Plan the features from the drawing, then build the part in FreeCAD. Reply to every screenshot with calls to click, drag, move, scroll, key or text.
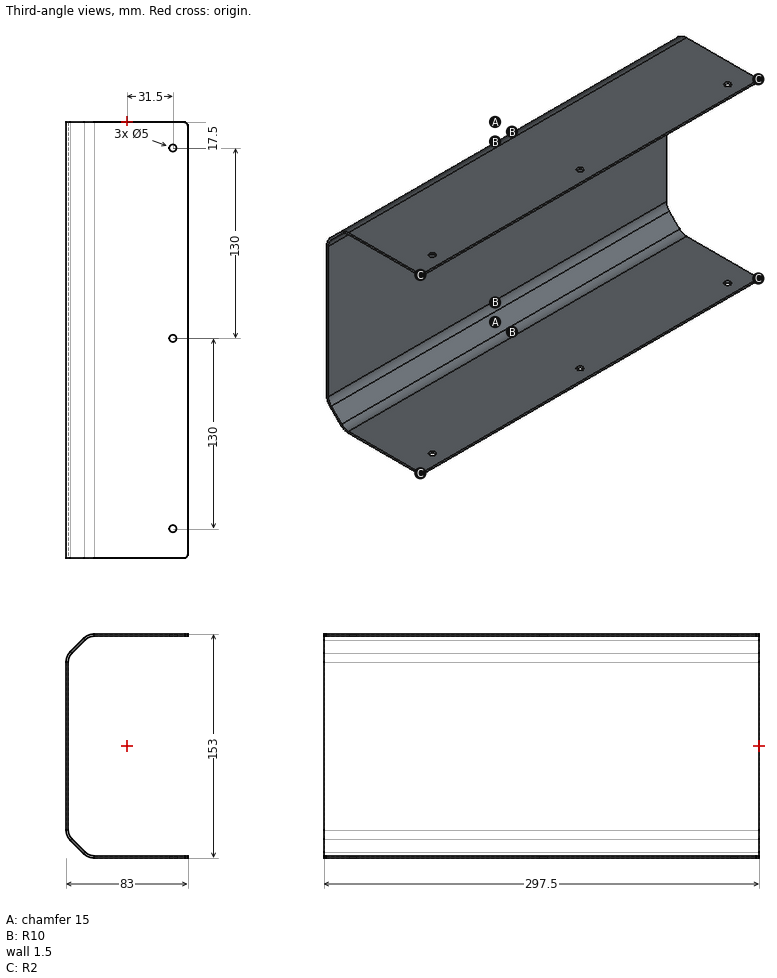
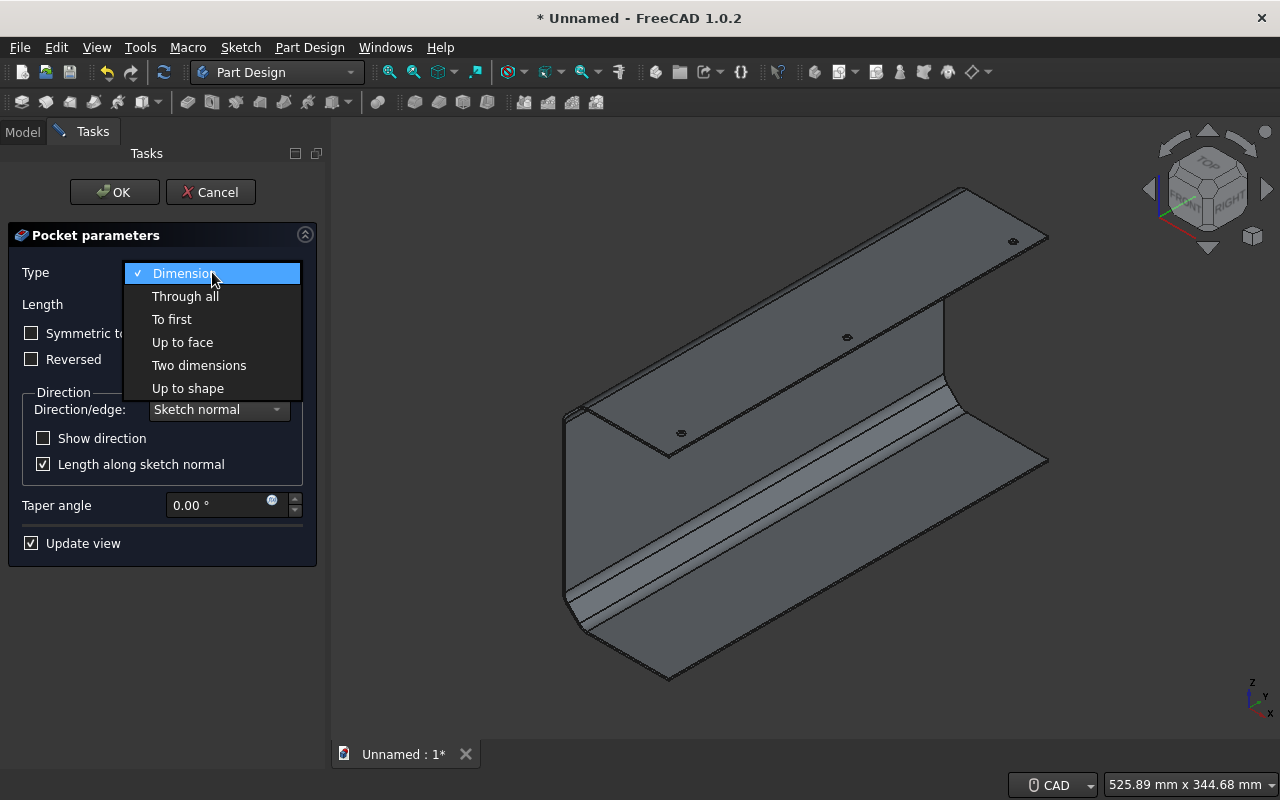
click(212, 296)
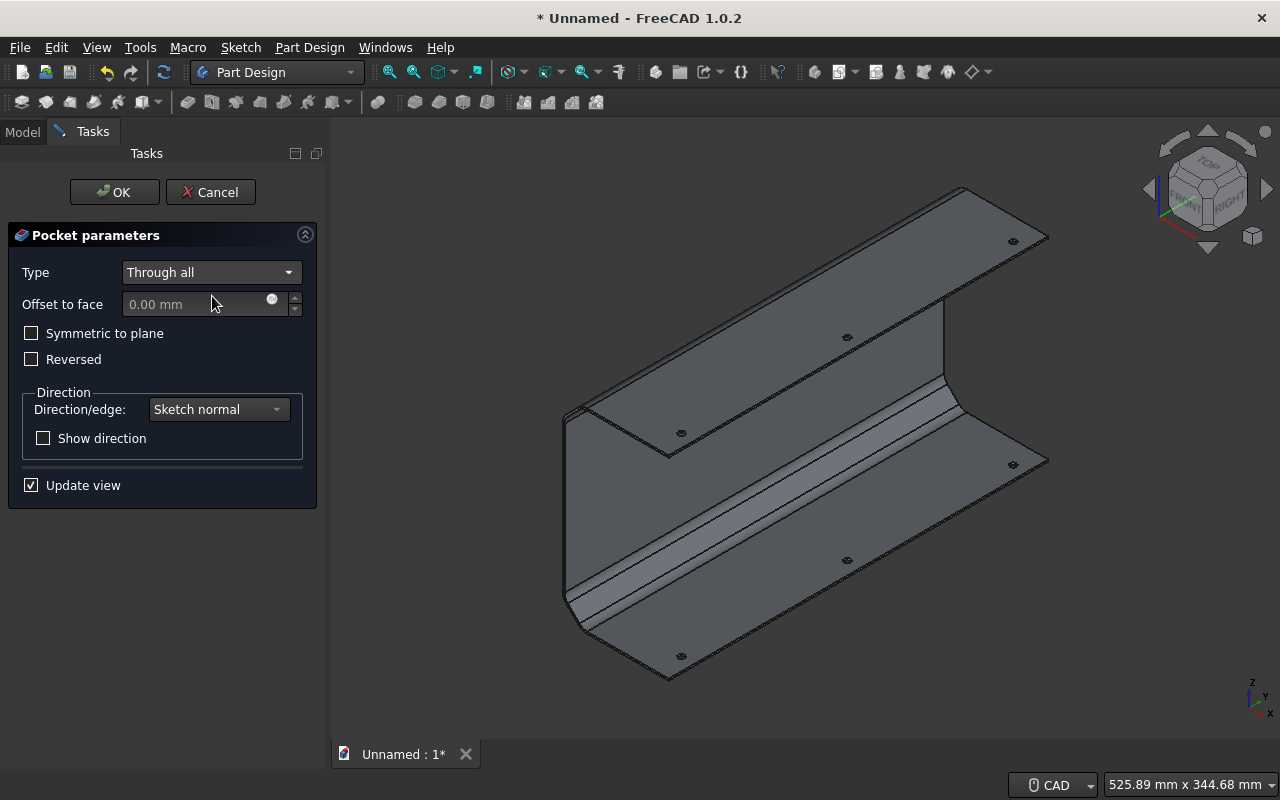
click(115, 192)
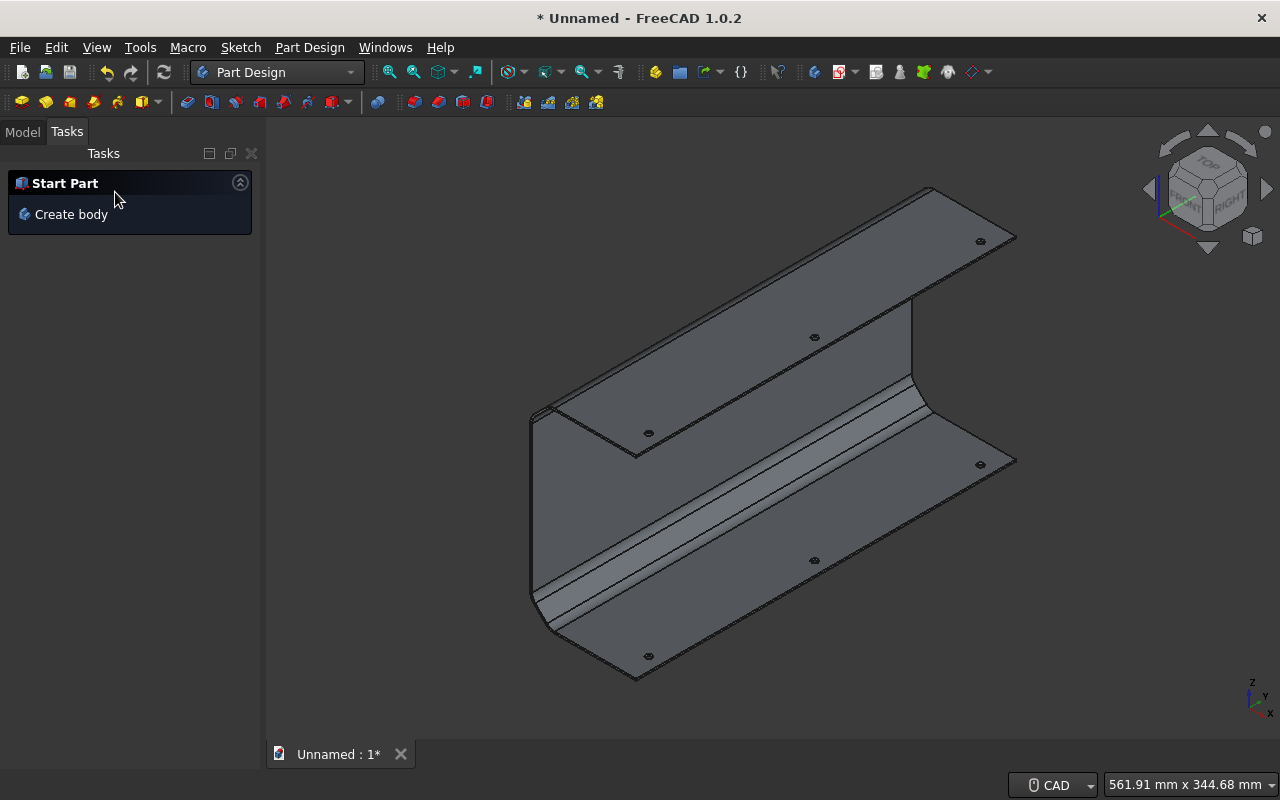
scroll(636, 456, up, 14)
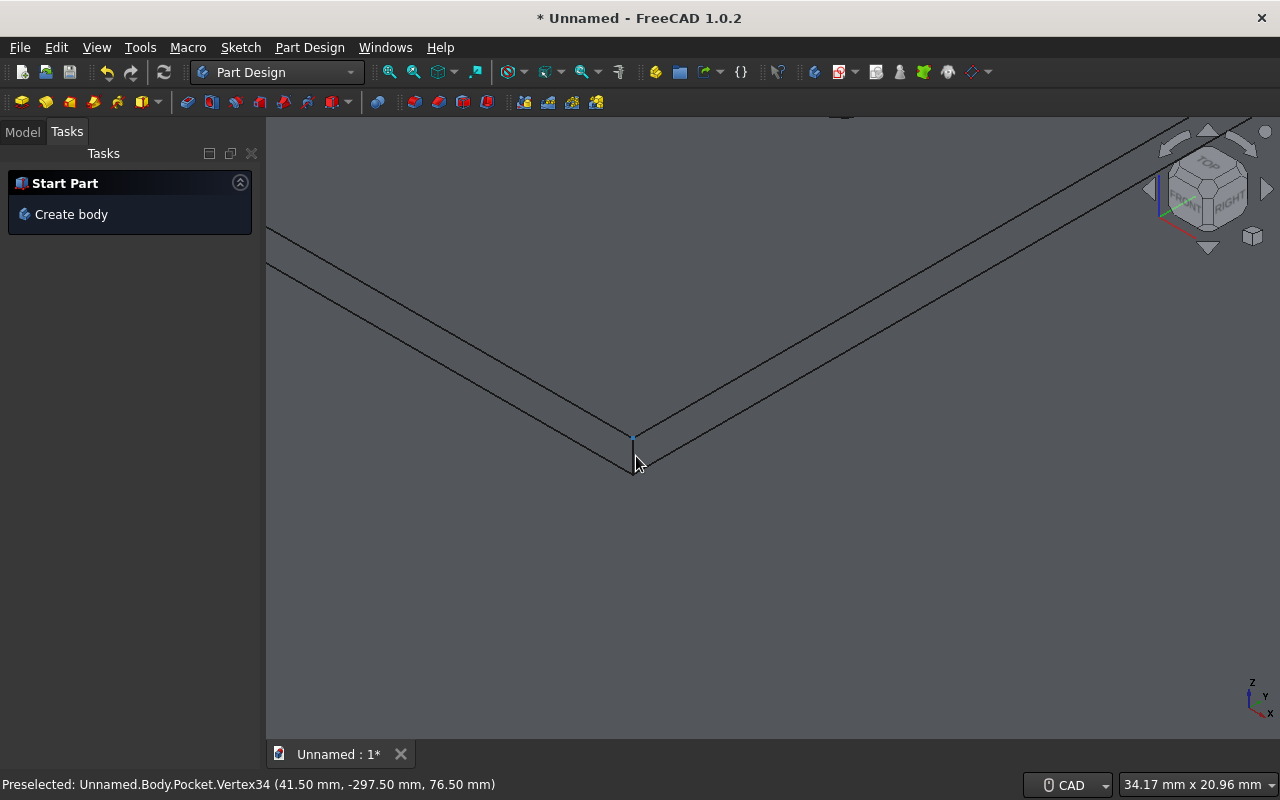
click(633, 456)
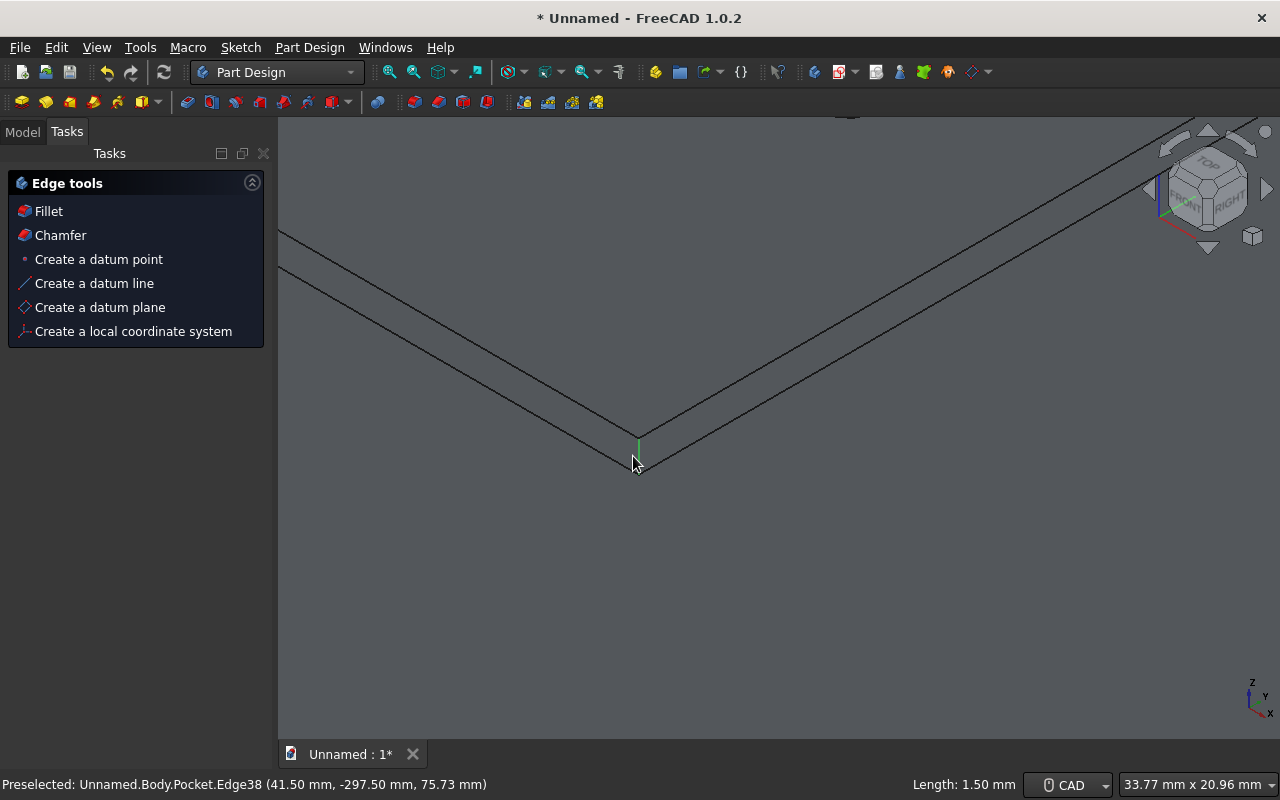
key(v)
key(f)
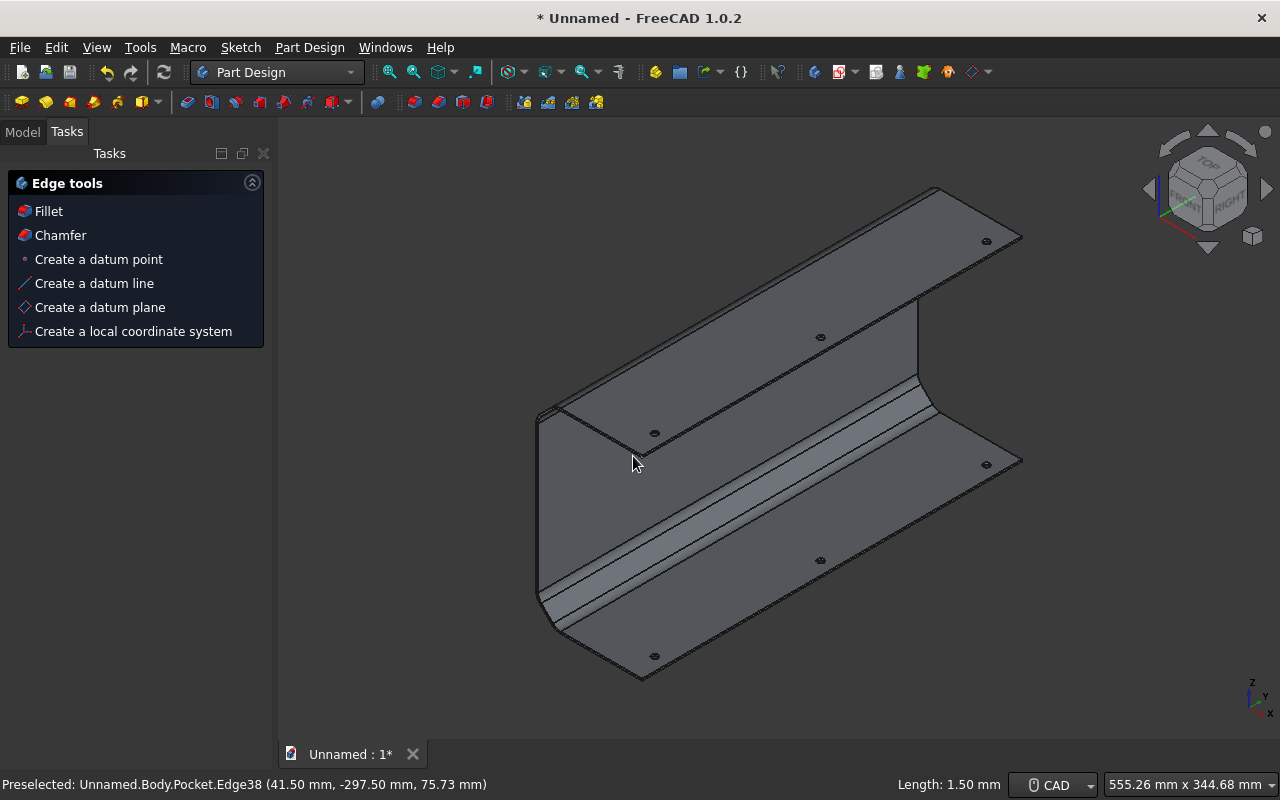
key(2)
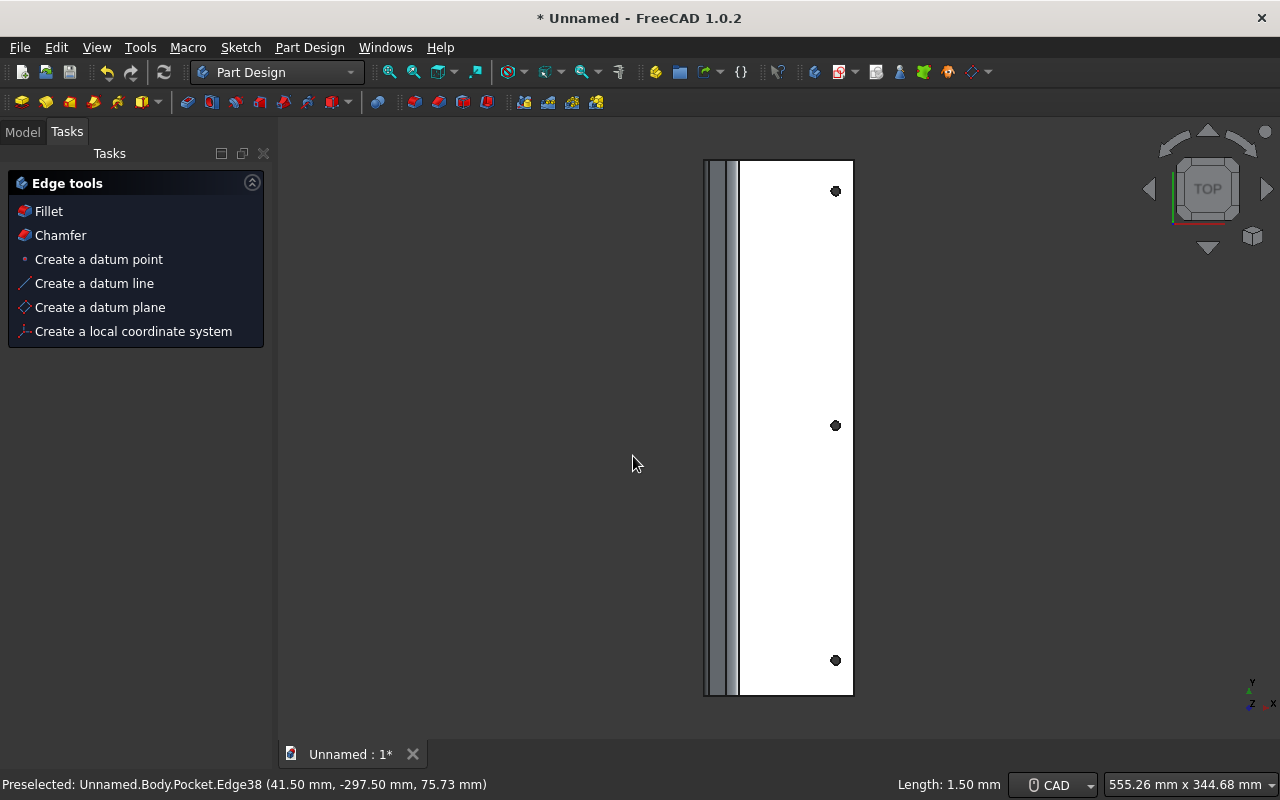
scroll(854, 159, up, 14)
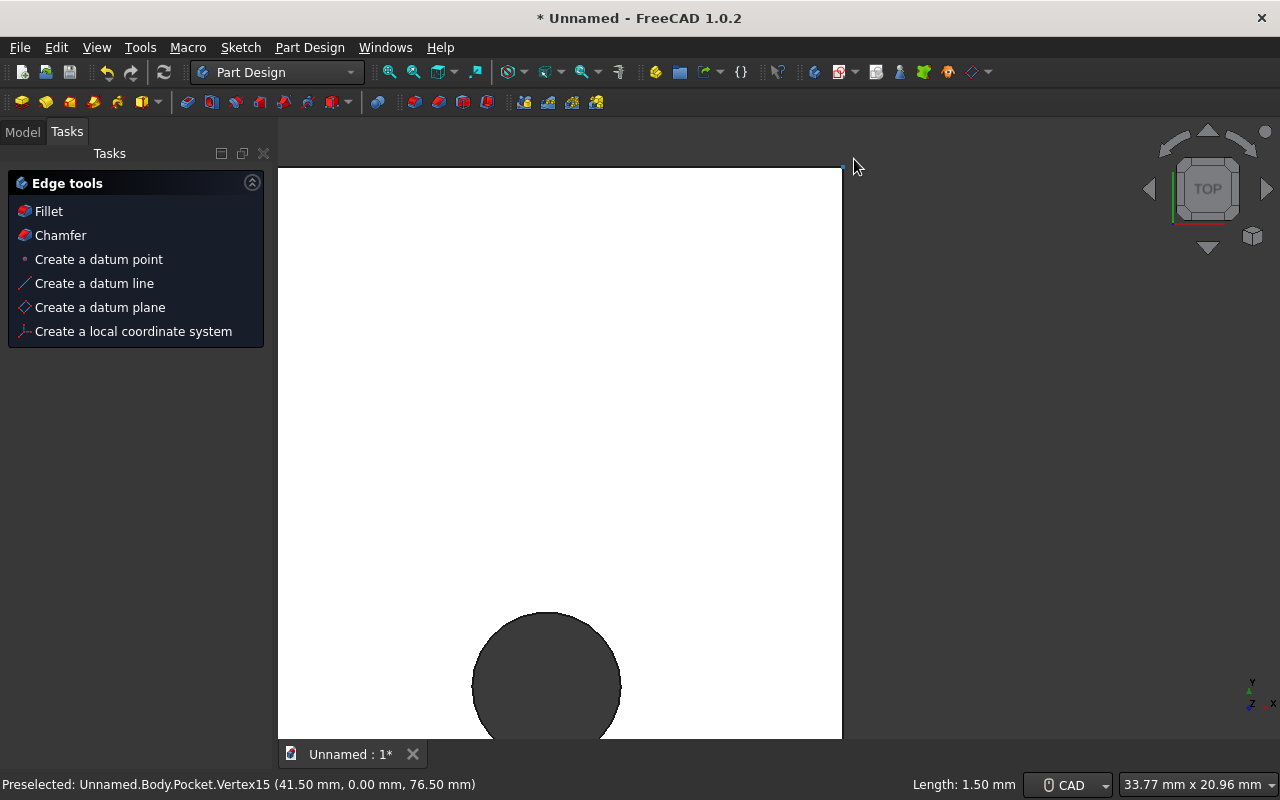
key(v)
key(f)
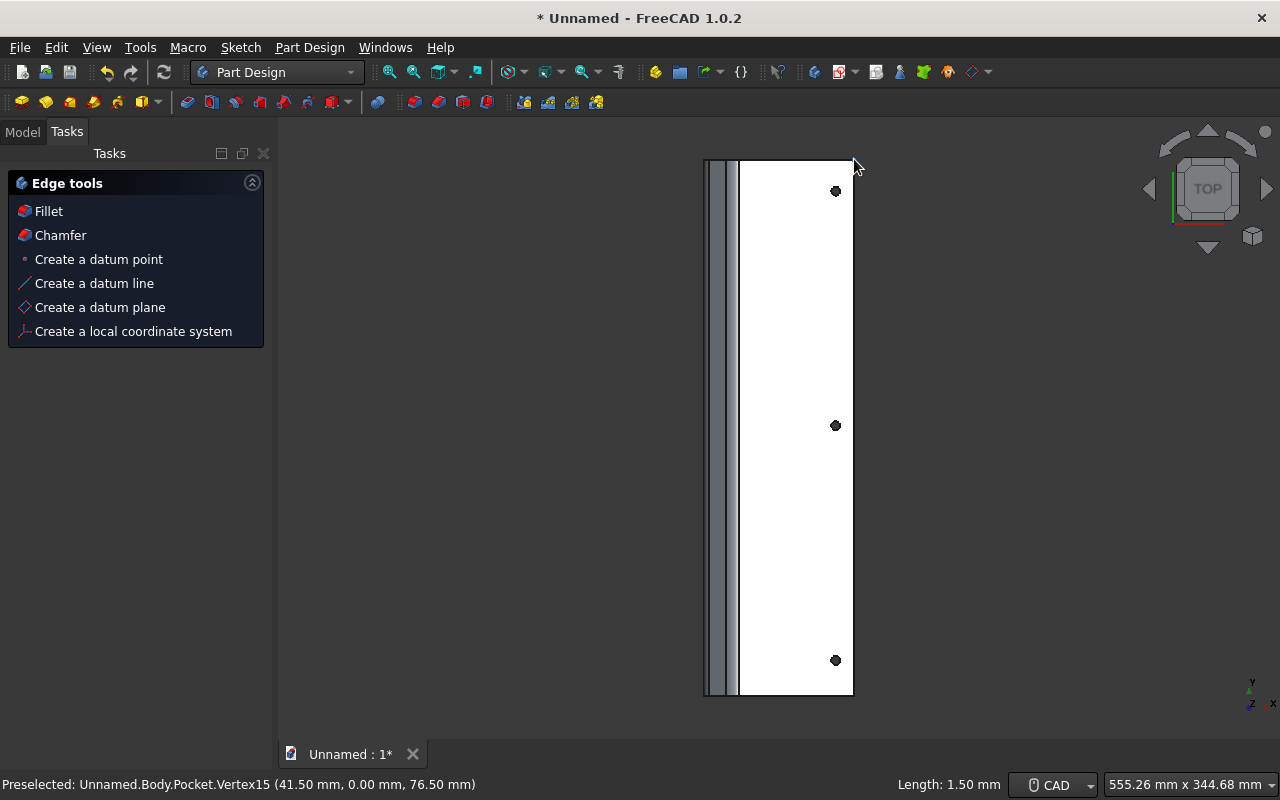
key(0)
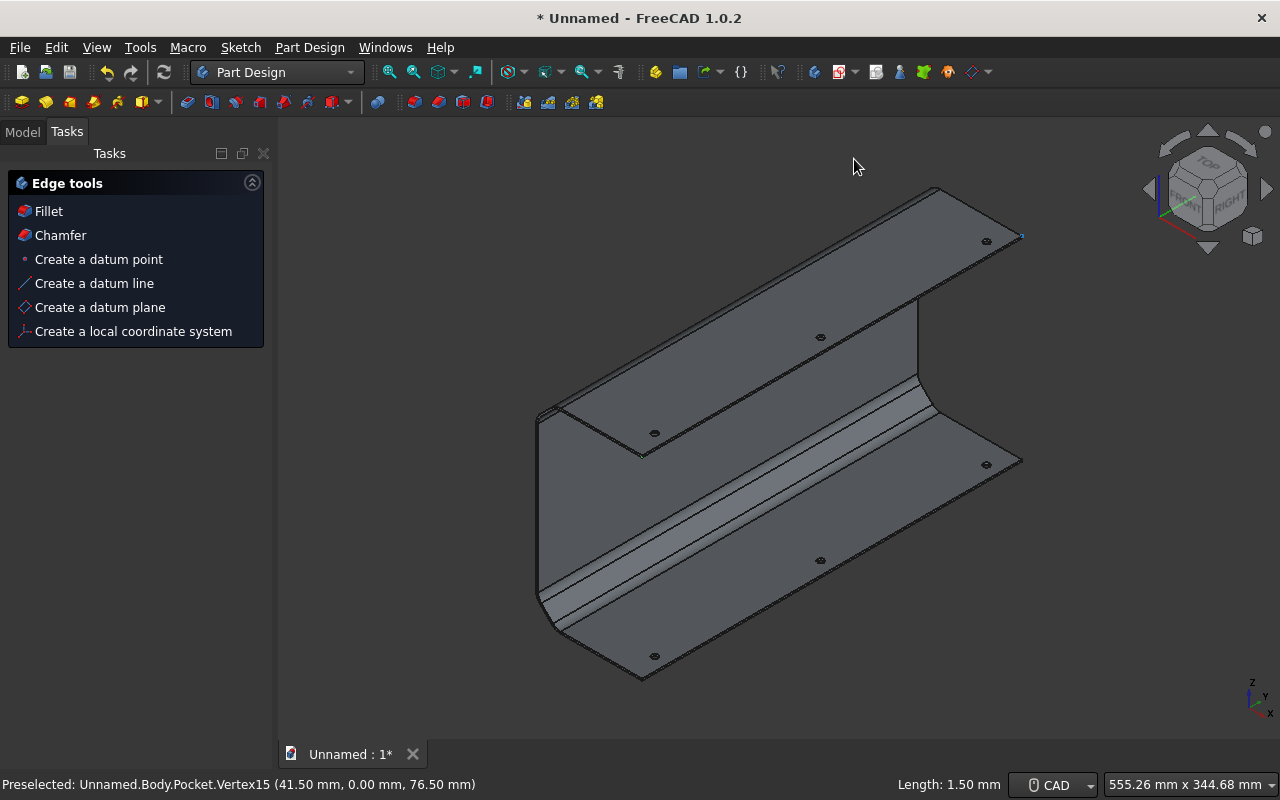
scroll(1022, 460, up, 14)